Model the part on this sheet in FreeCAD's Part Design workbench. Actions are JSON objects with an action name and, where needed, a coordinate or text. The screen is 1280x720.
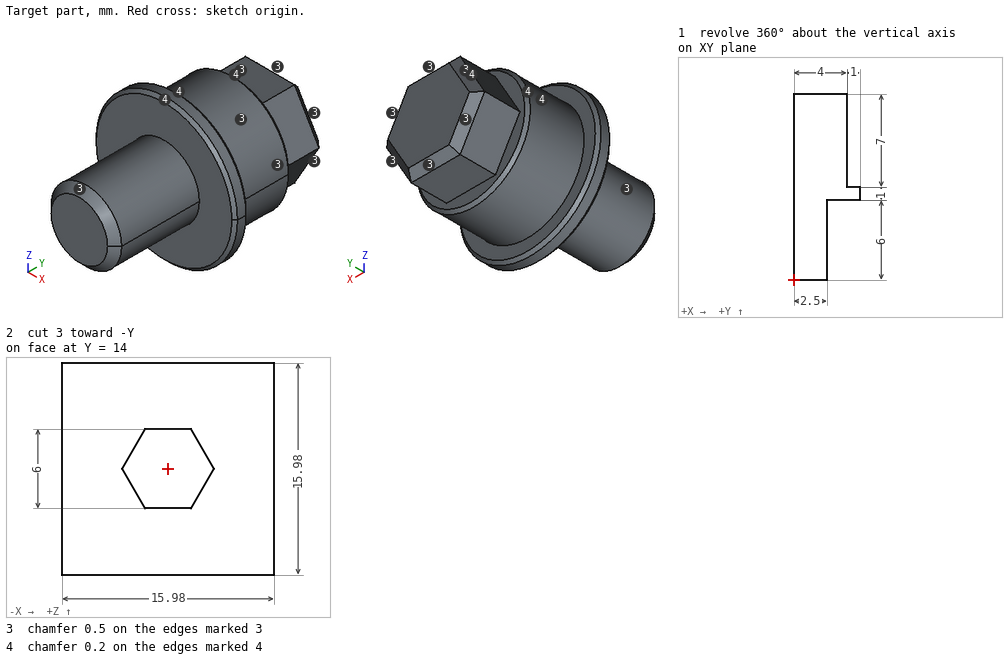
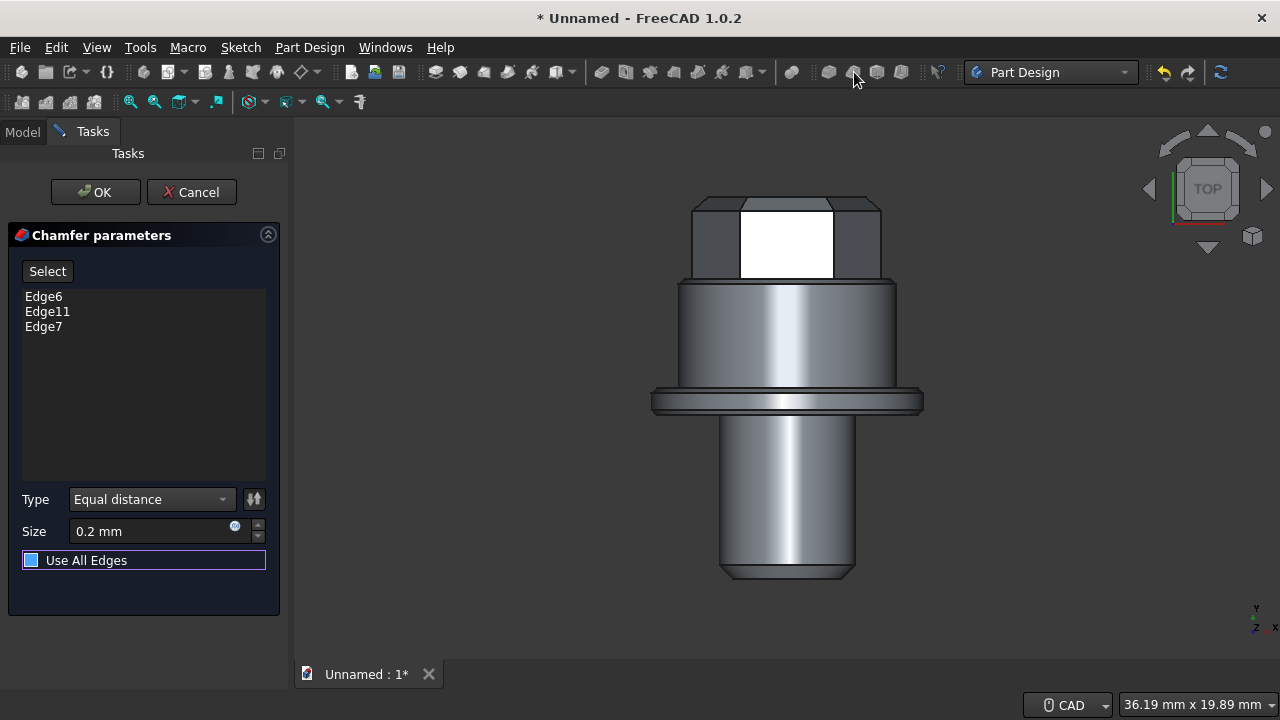
{"action": "left_click", "coordinate": [96, 192]}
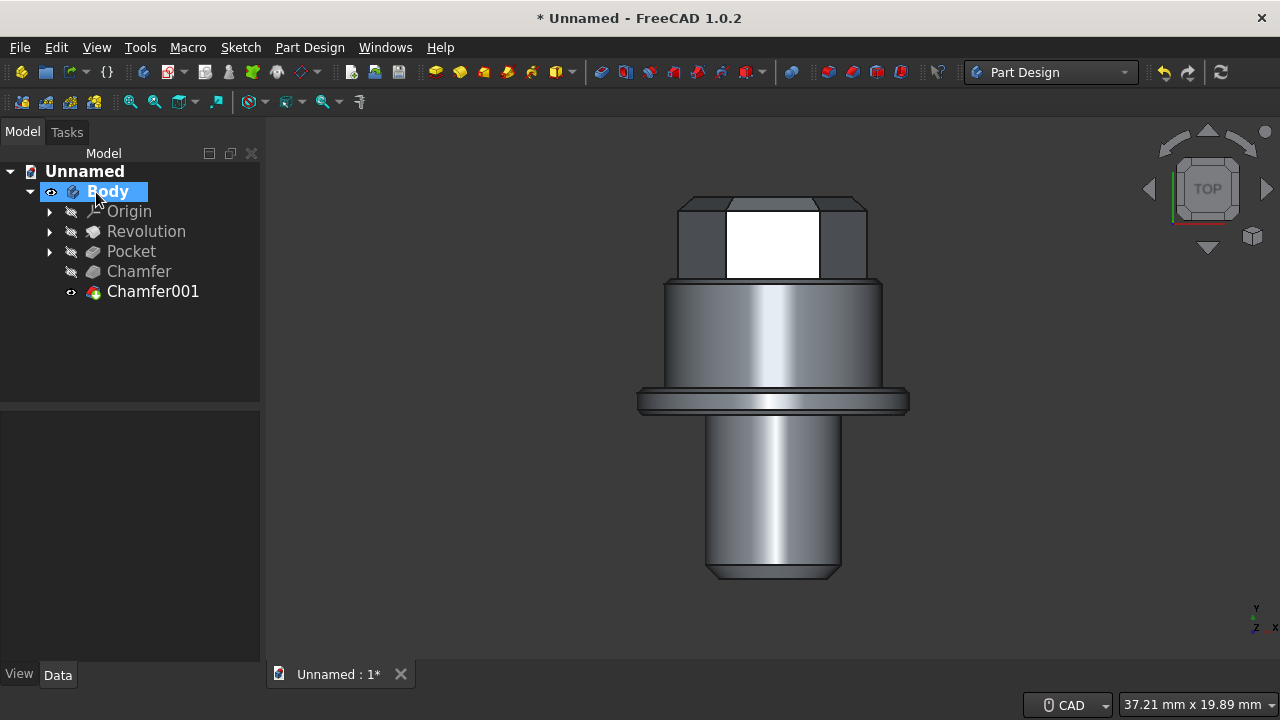
{"action": "key", "text": "0"}